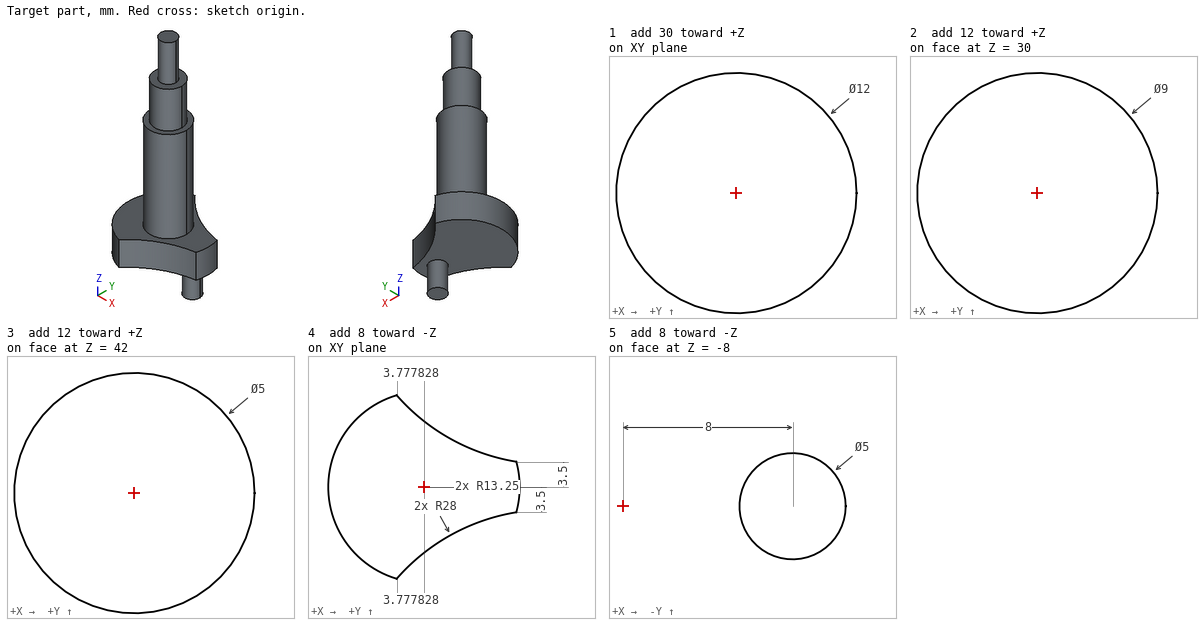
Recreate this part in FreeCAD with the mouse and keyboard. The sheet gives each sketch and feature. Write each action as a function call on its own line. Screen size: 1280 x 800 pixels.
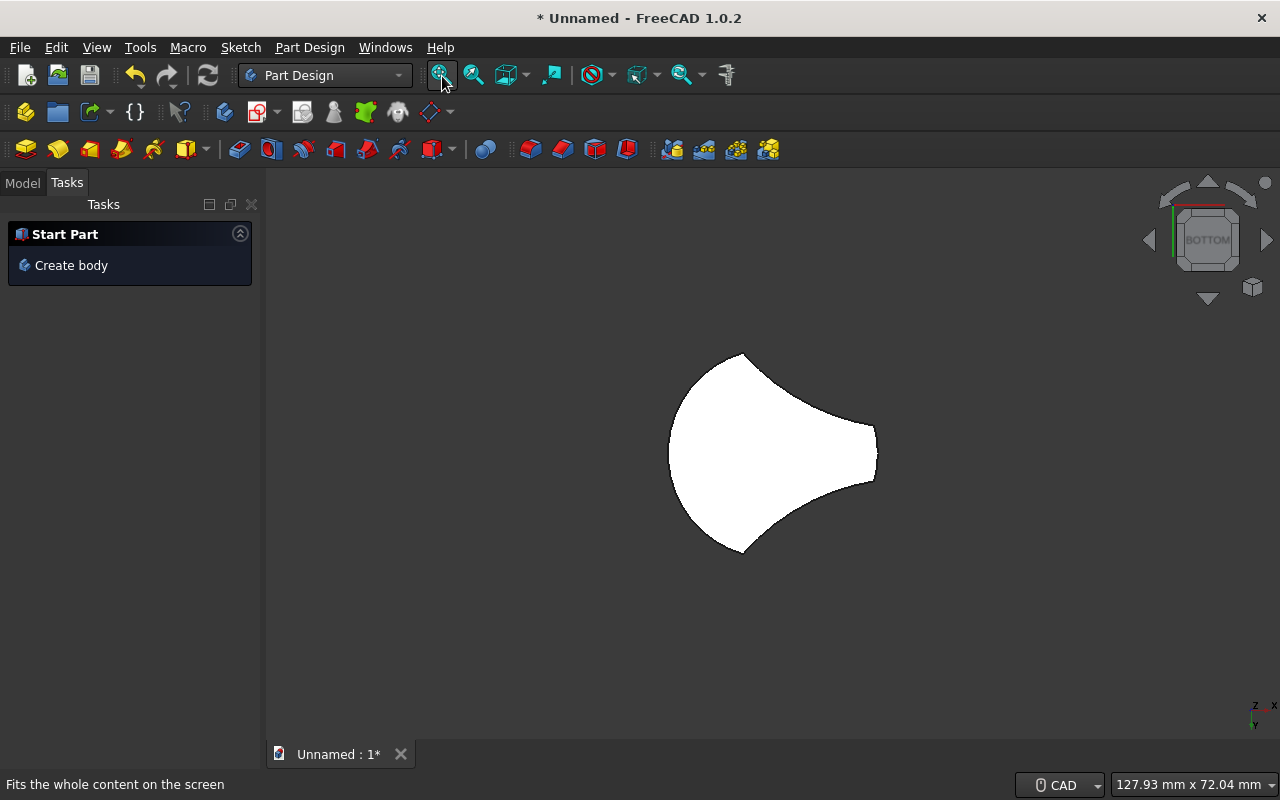
click(442, 76)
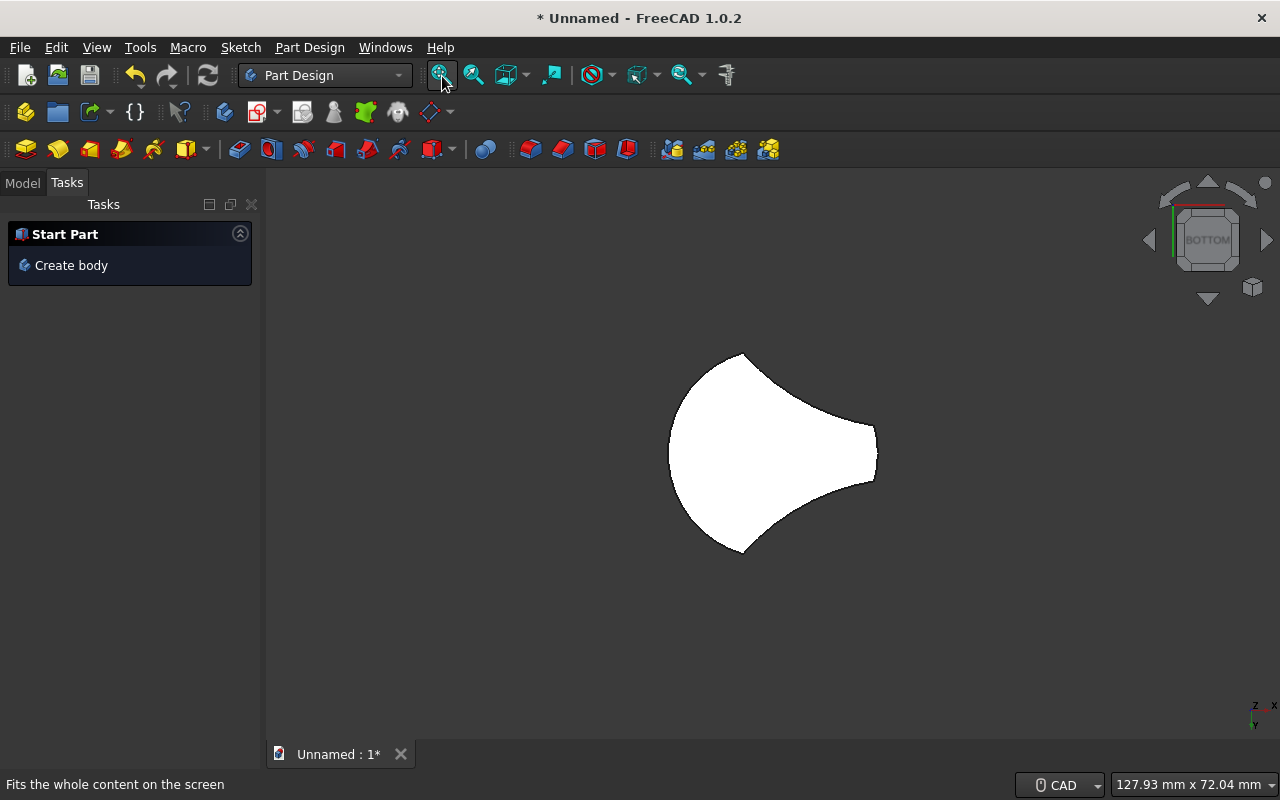
click(743, 452)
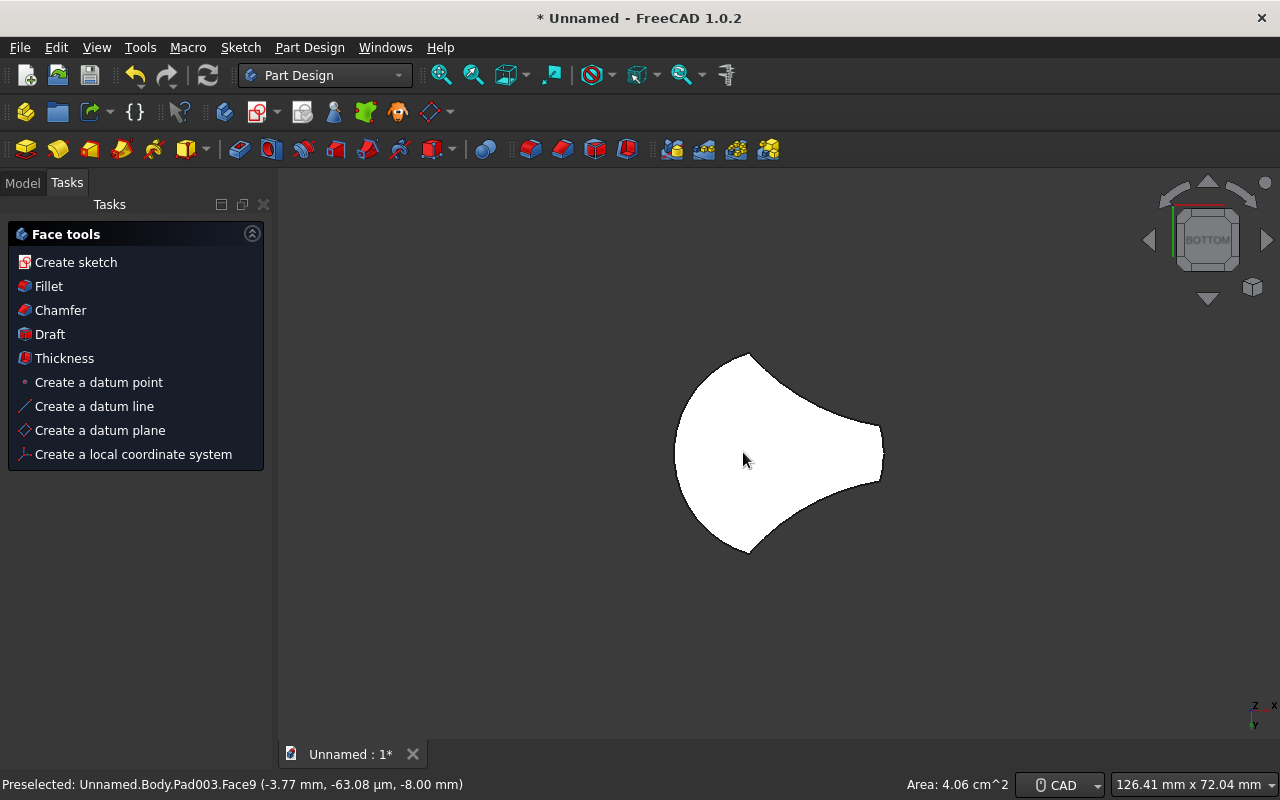
click(258, 112)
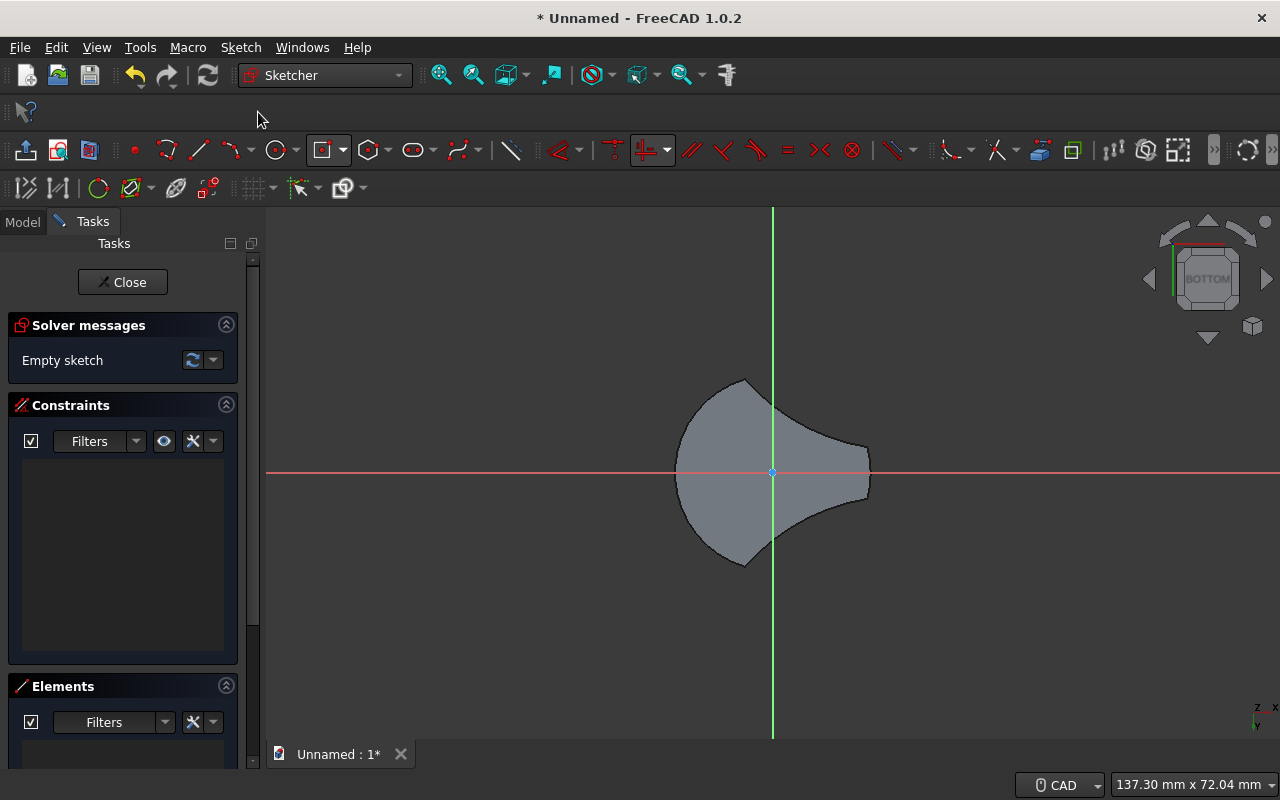
scroll(828, 473, up, 10)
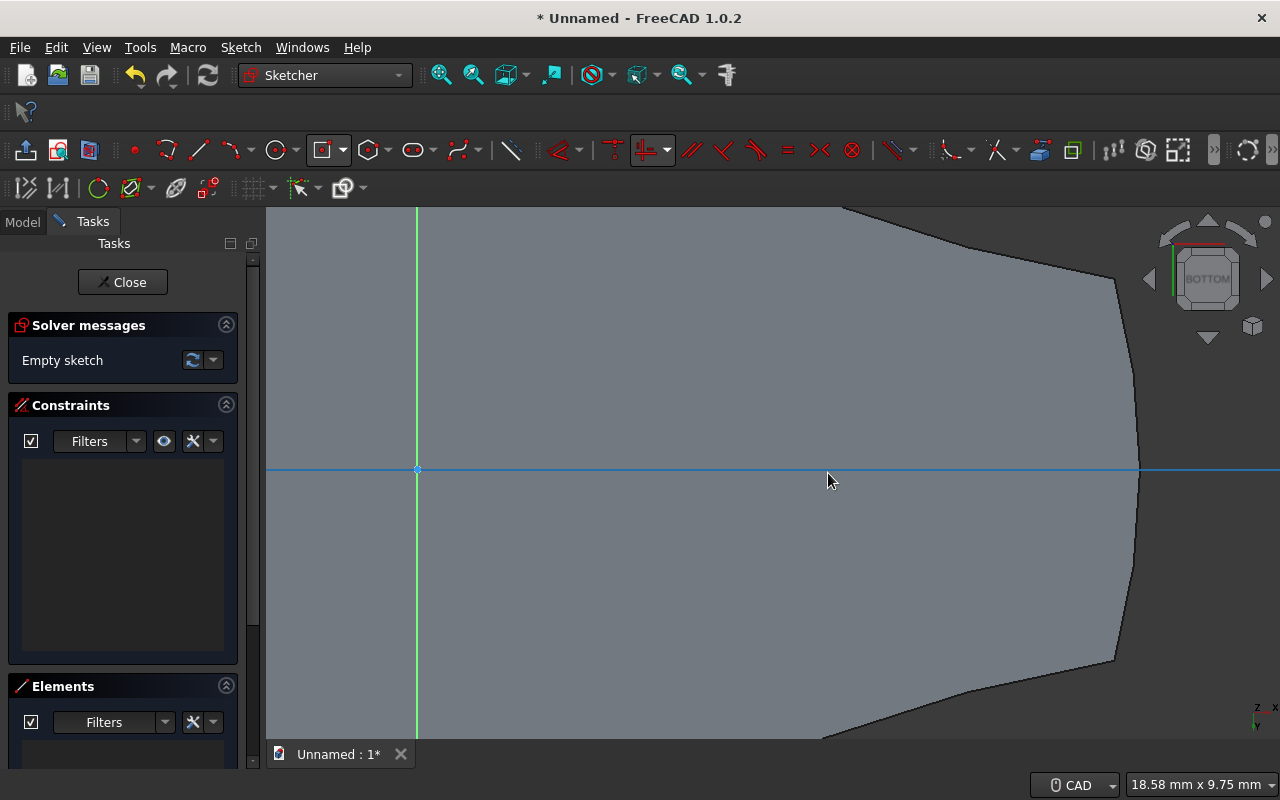
click(276, 150)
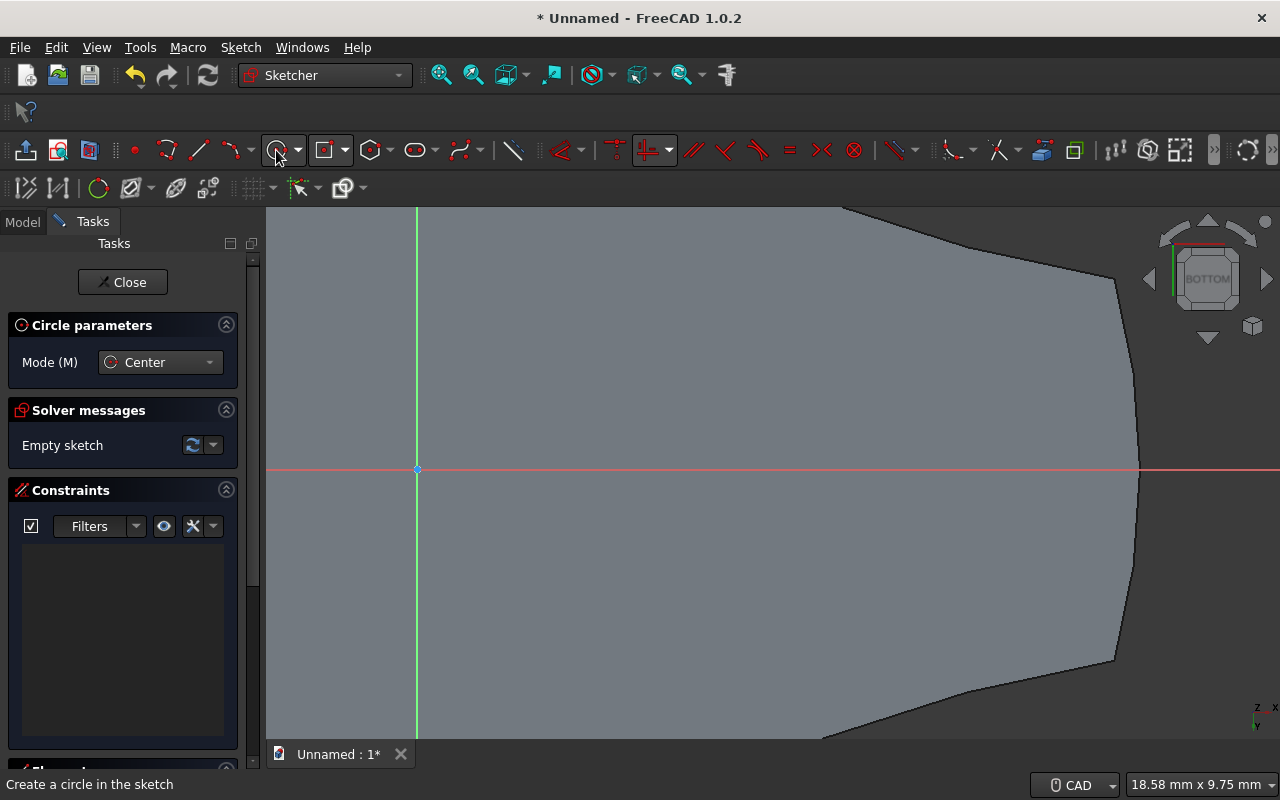
click(854, 470)
move(950, 373)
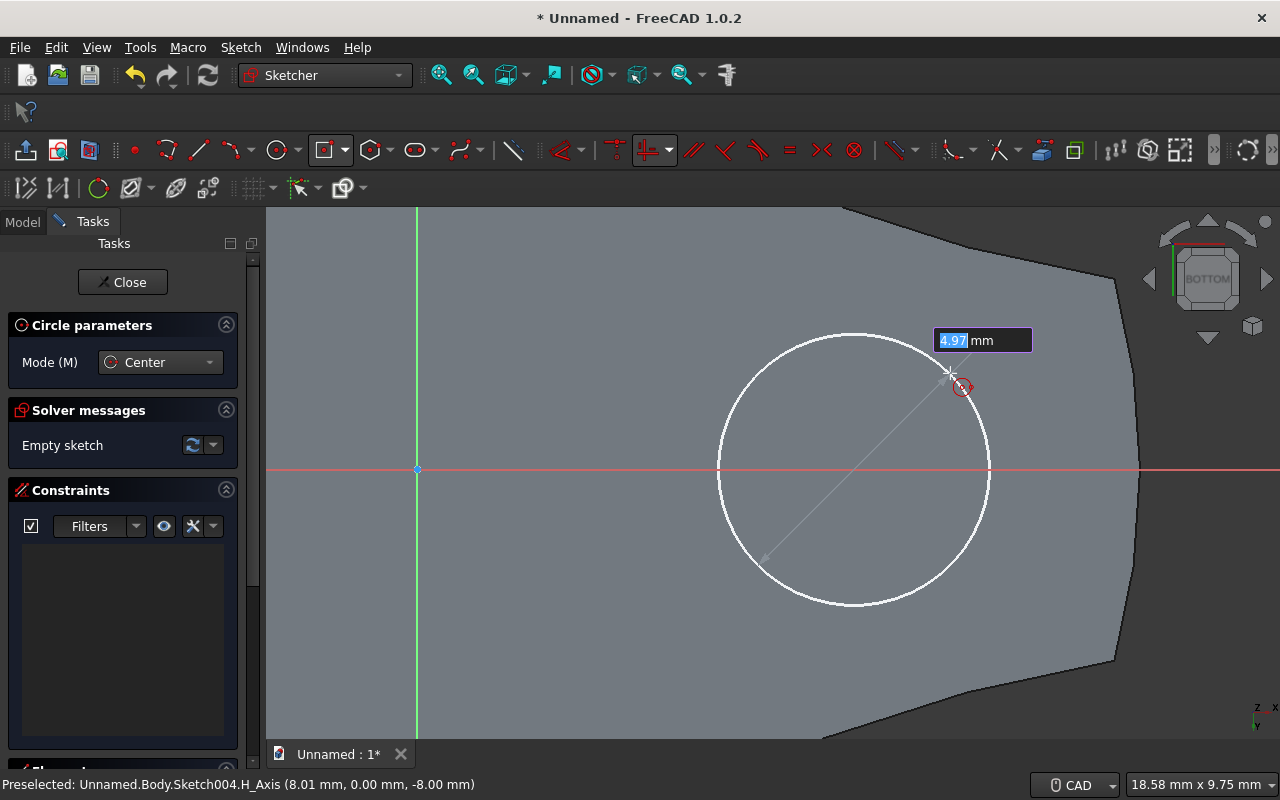
text(5)
key(Return)
key(Escape)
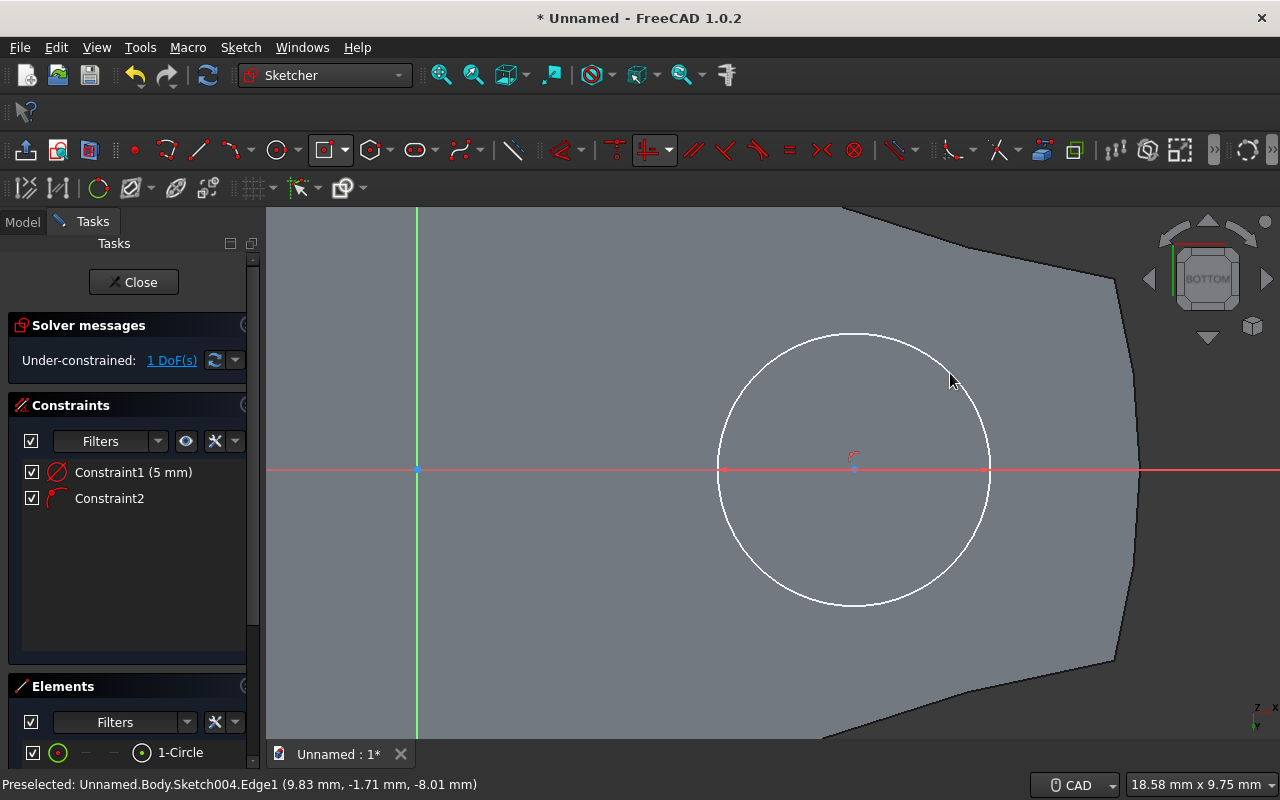
click(560, 150)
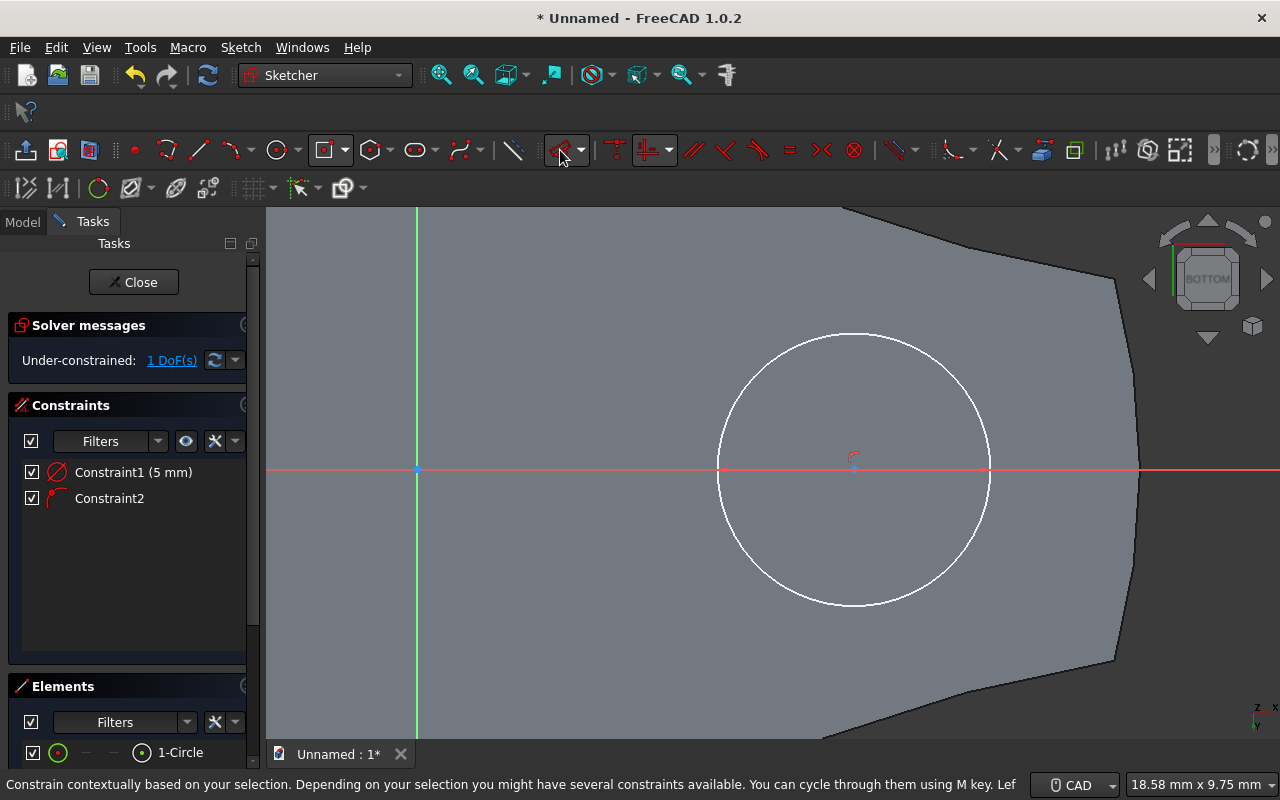
click(854, 470)
click(636, 504)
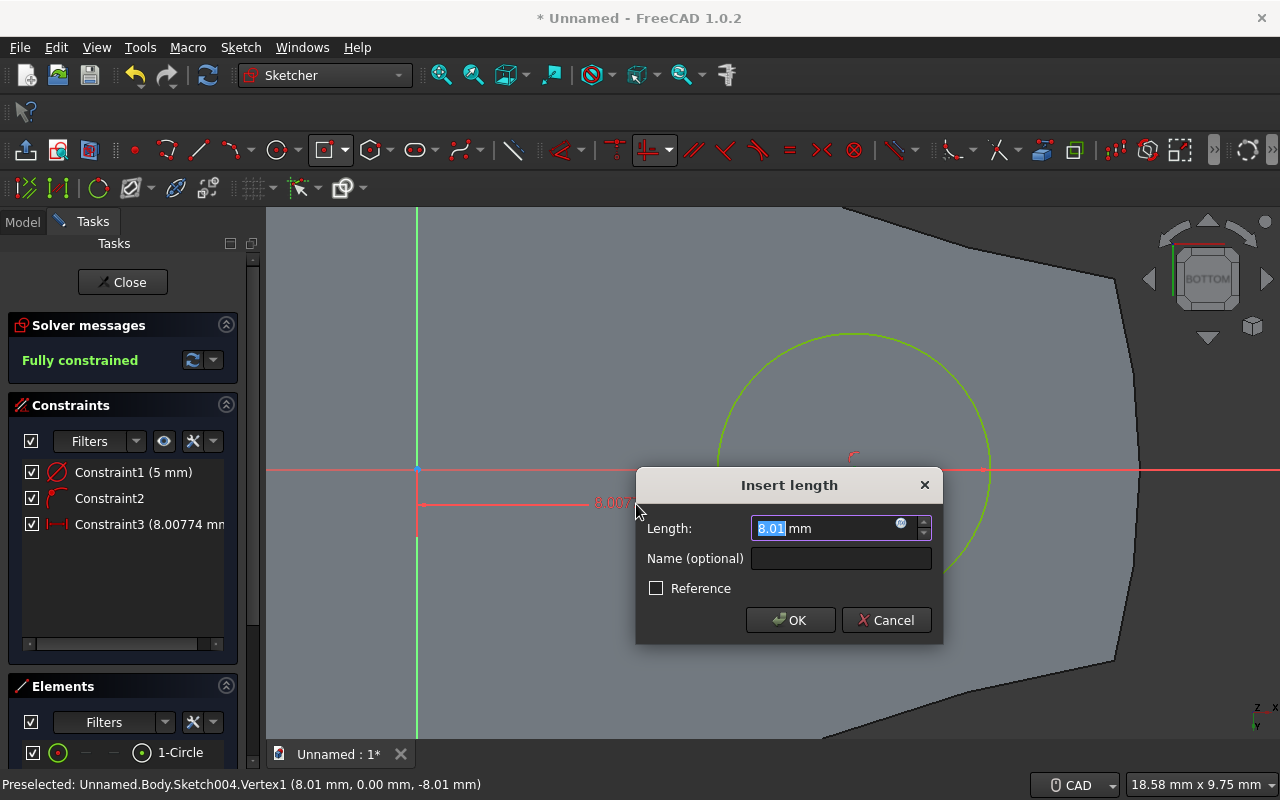
text(8)
key(Return)
key(Escape)